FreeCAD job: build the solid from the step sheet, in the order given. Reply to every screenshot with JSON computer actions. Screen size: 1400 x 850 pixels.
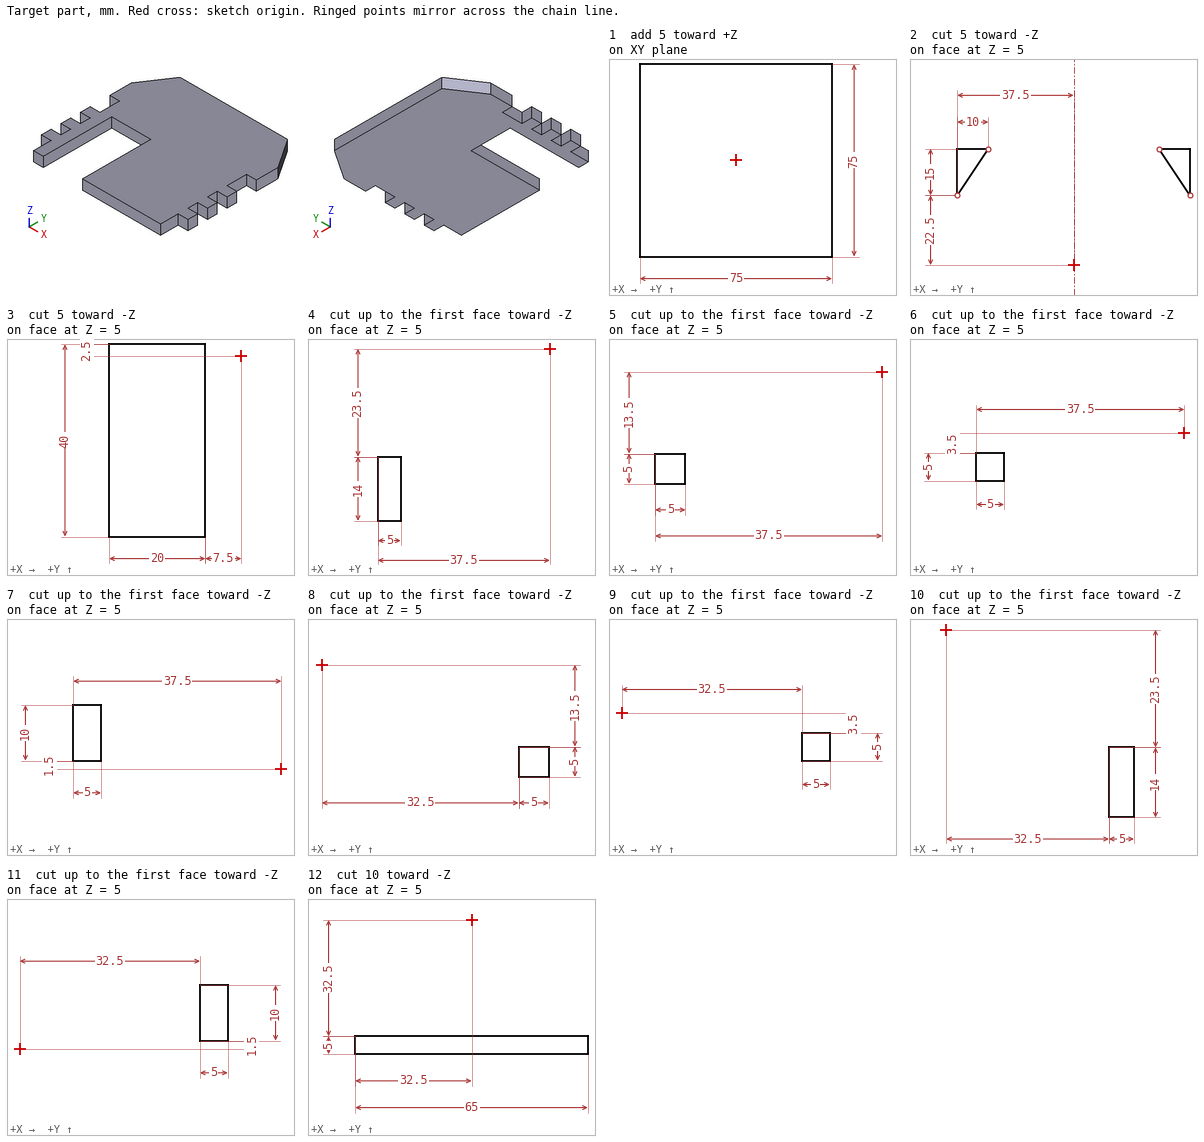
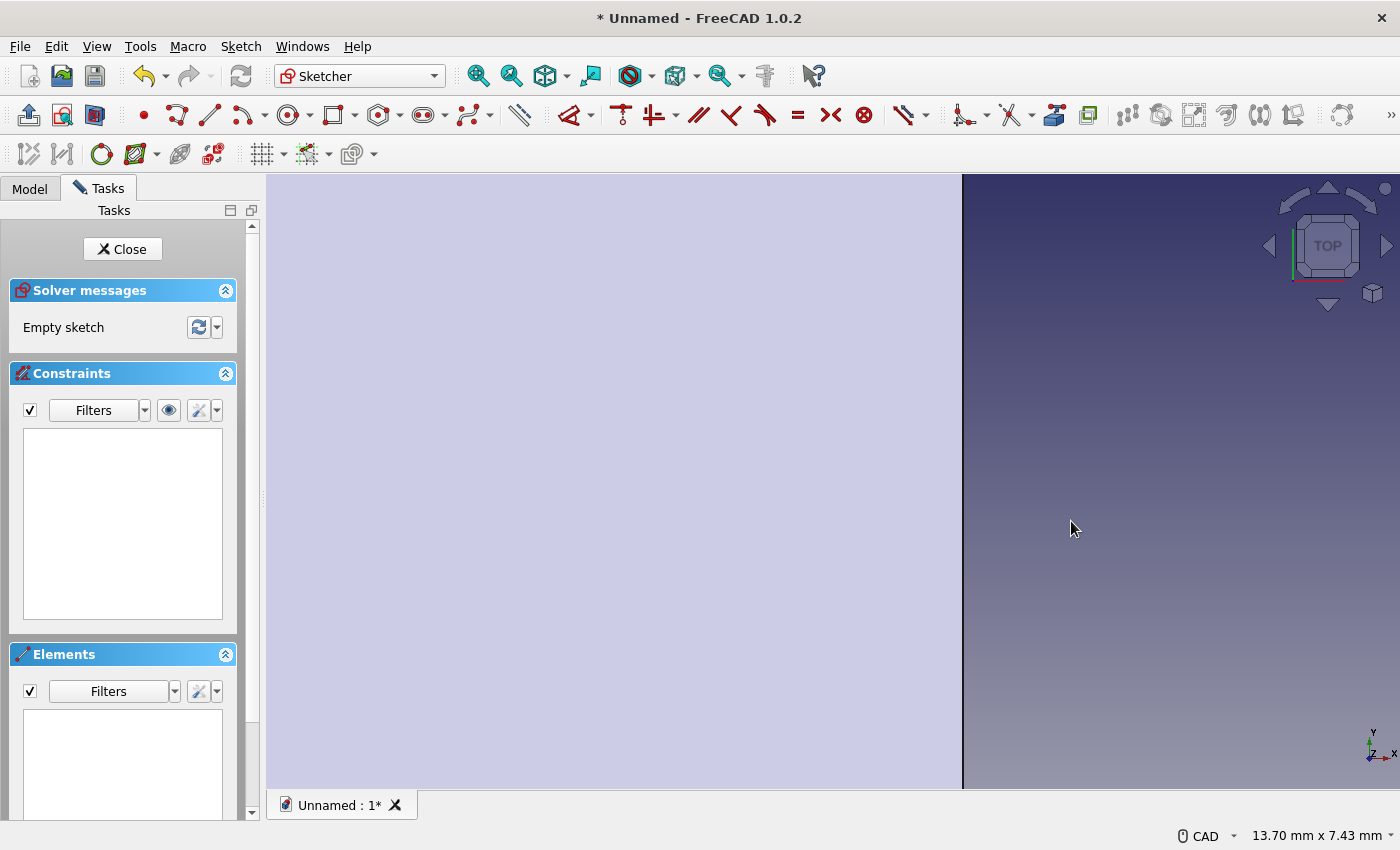
{"action": "key", "text": "g r"}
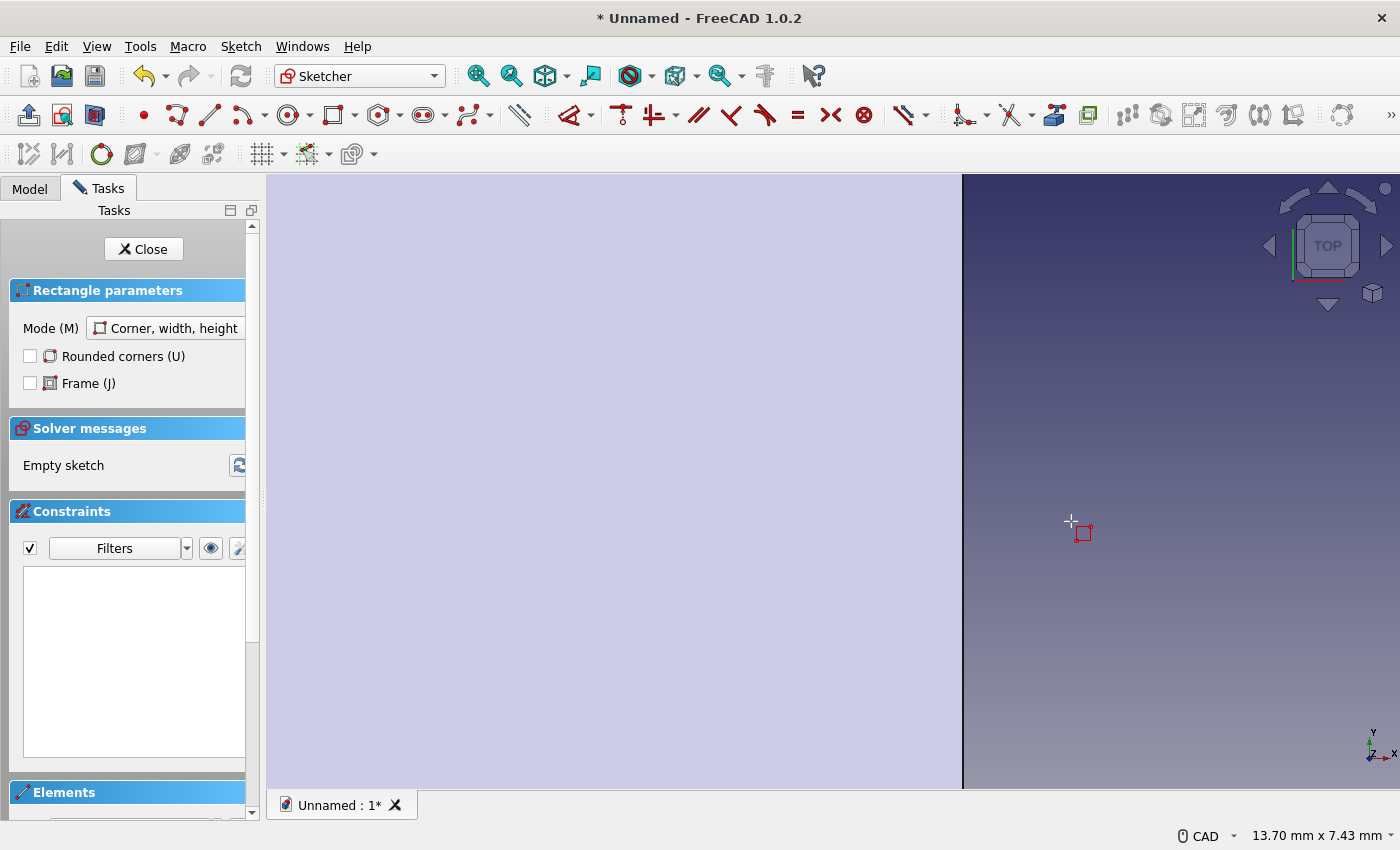
{"action": "left_click", "coordinate": [549, 272]}
{"action": "left_click", "coordinate": [963, 686]}
{"action": "key", "text": "Escape"}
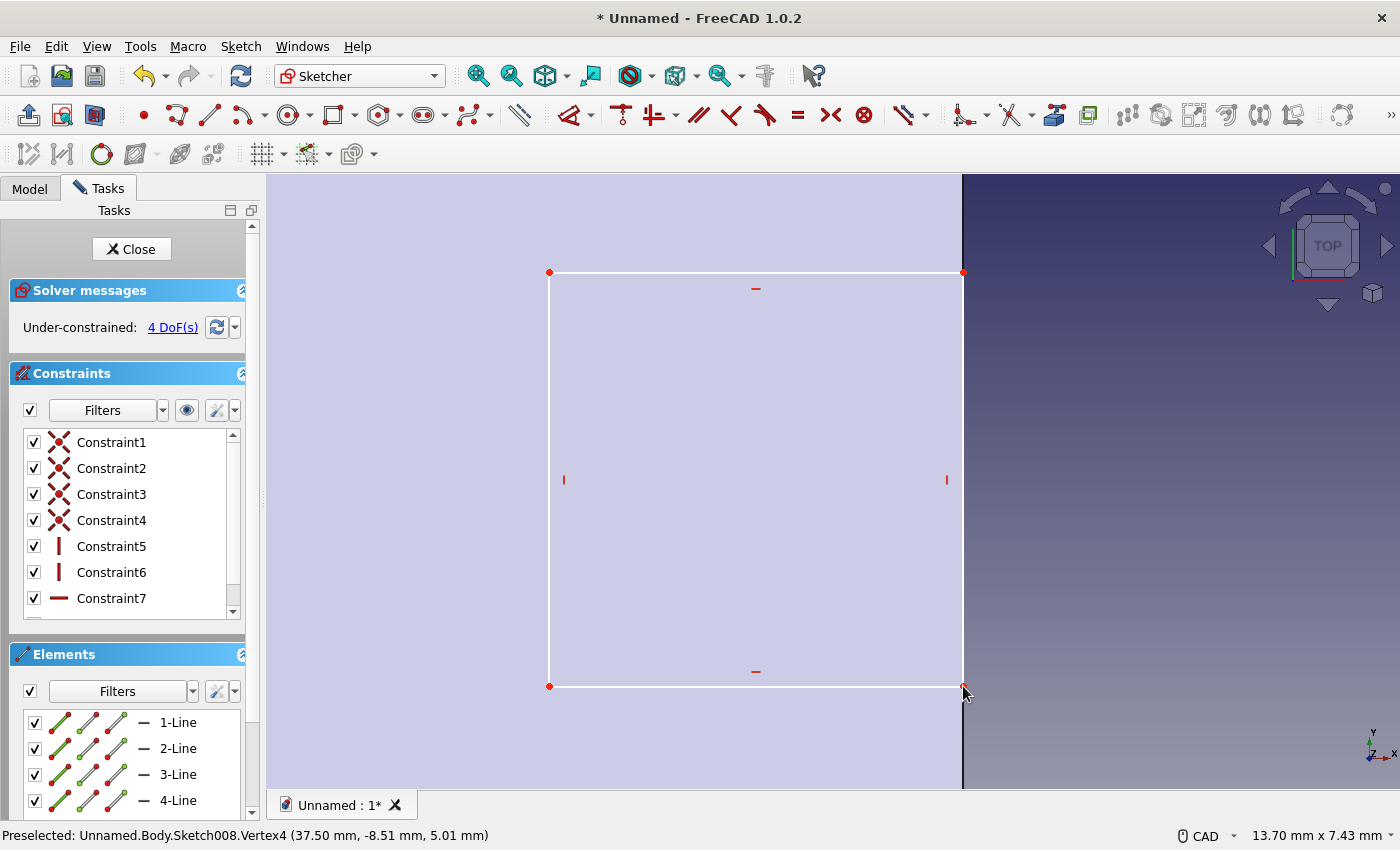
{"action": "left_click", "coordinate": [568, 116]}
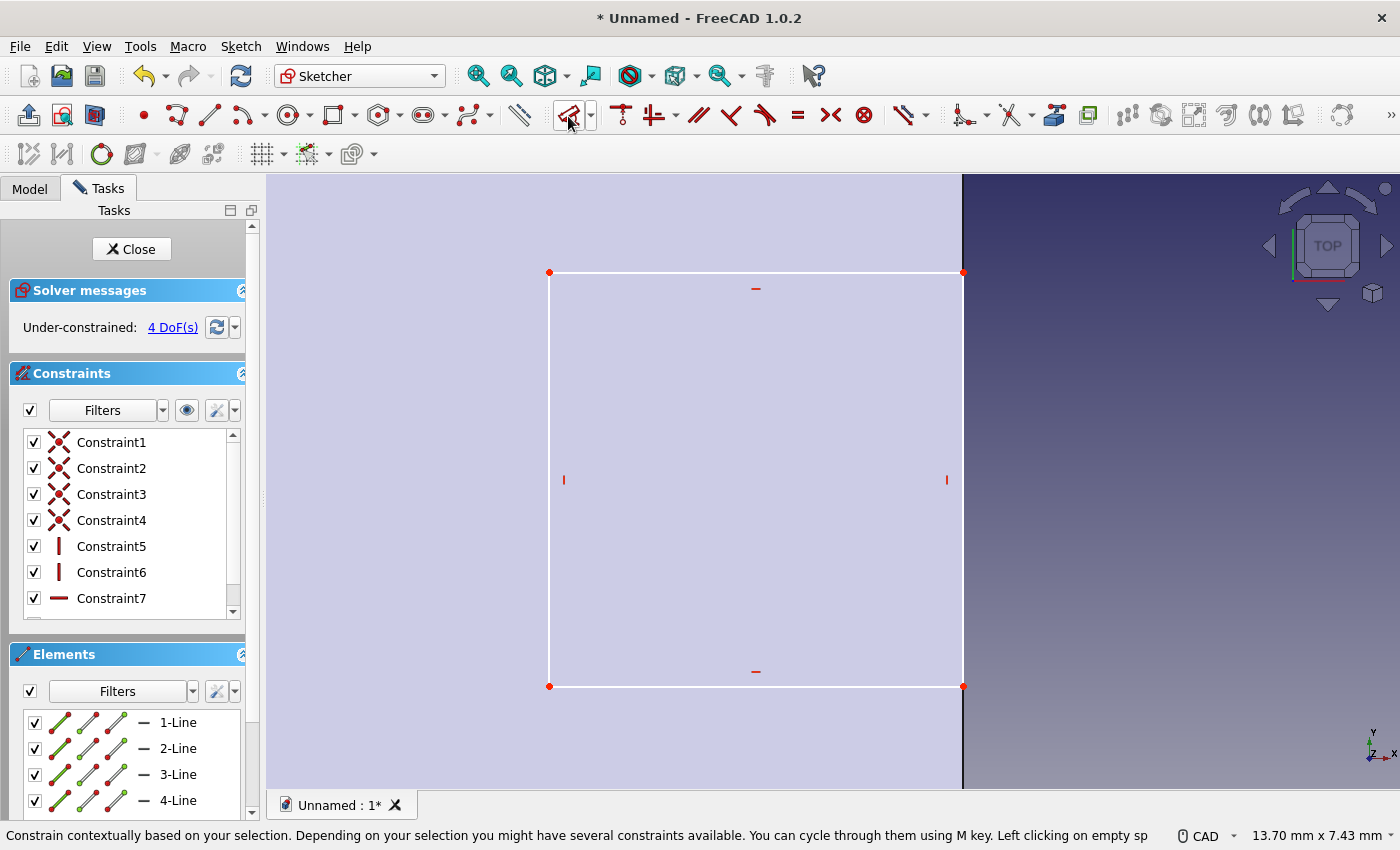
{"action": "left_click", "coordinate": [549, 397]}
{"action": "left_click", "coordinate": [515, 480]}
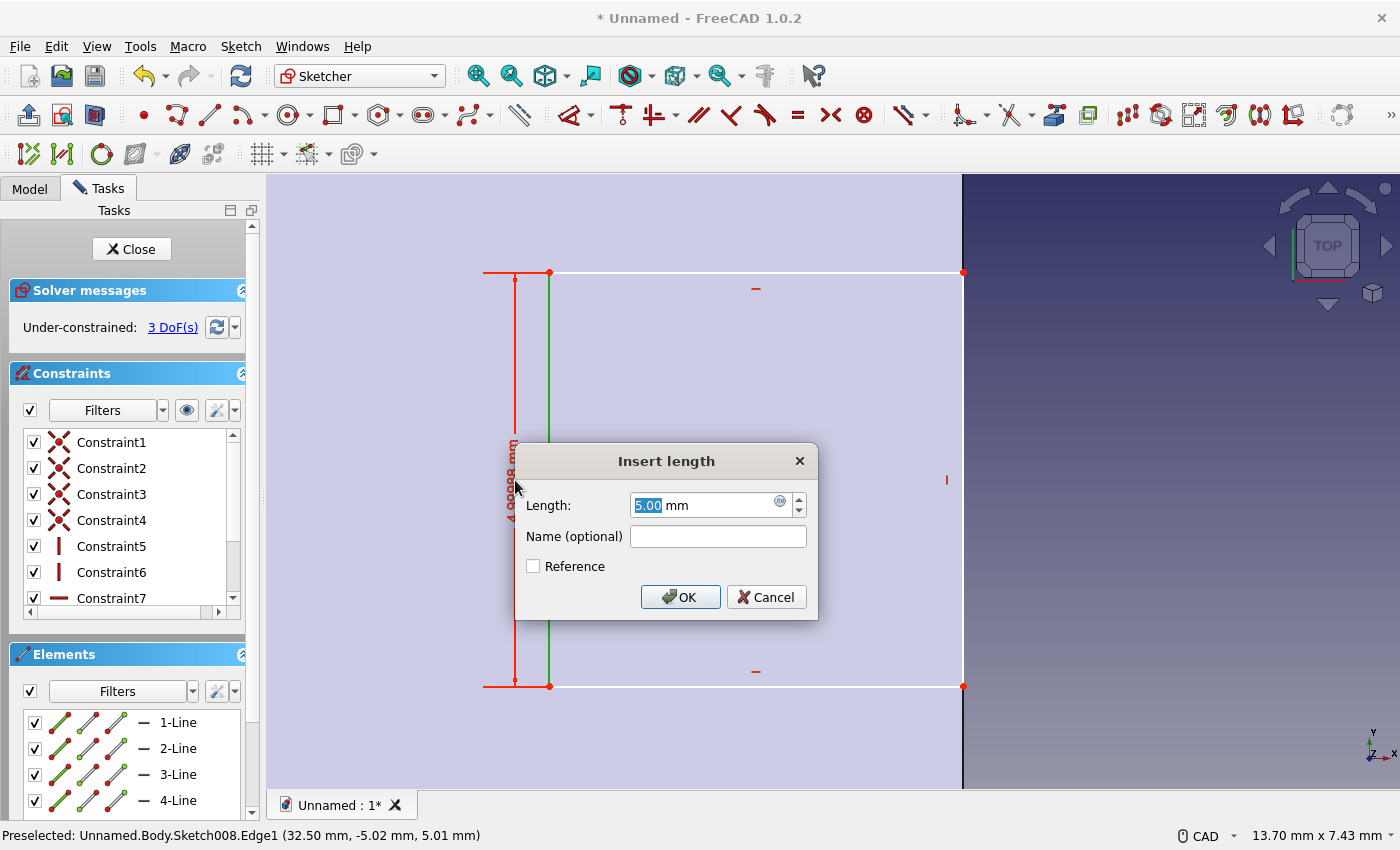
{"action": "type", "text": "5"}
{"action": "key", "text": "Return"}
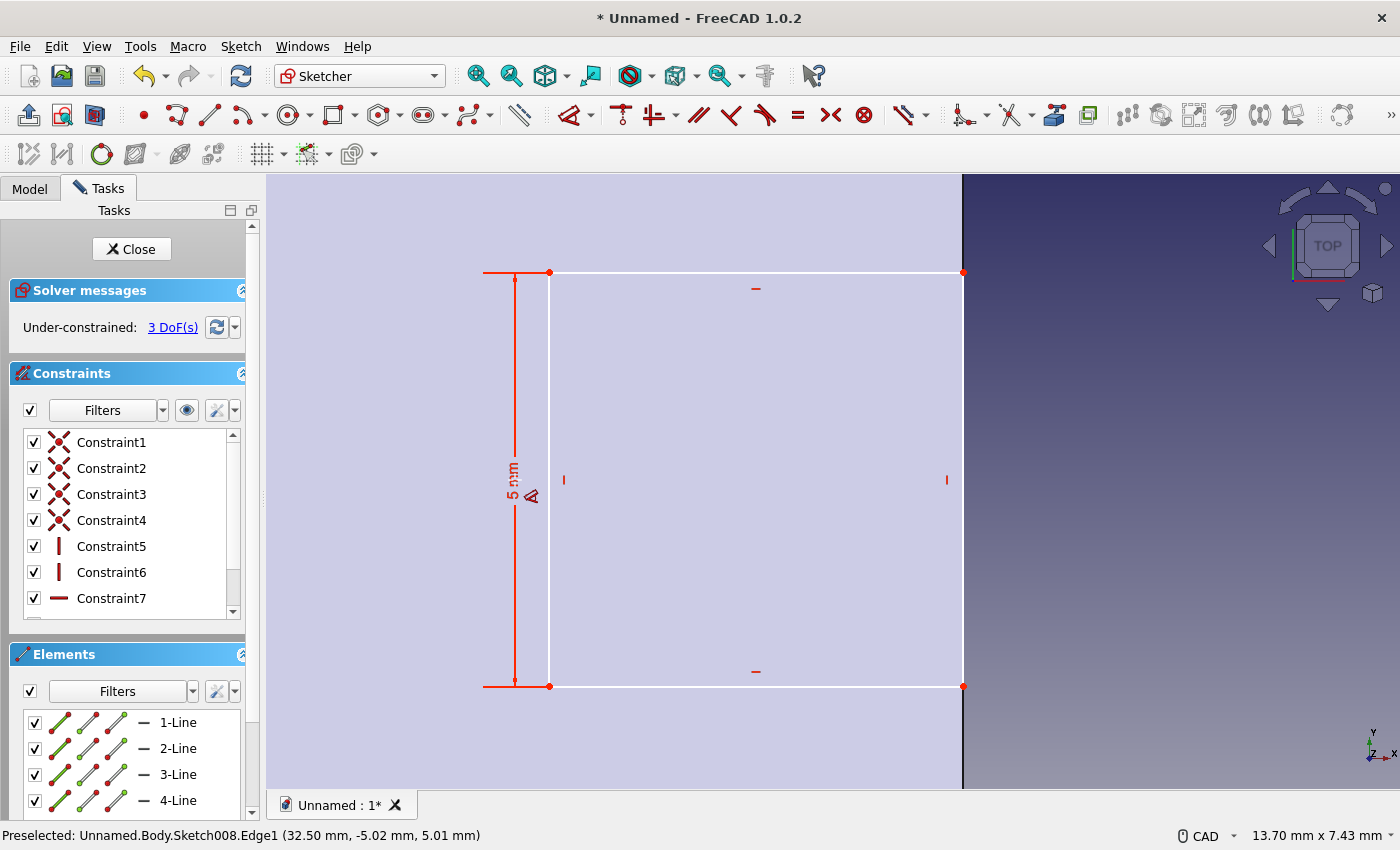
{"action": "left_click", "coordinate": [673, 687]}
{"action": "left_click", "coordinate": [756, 721]}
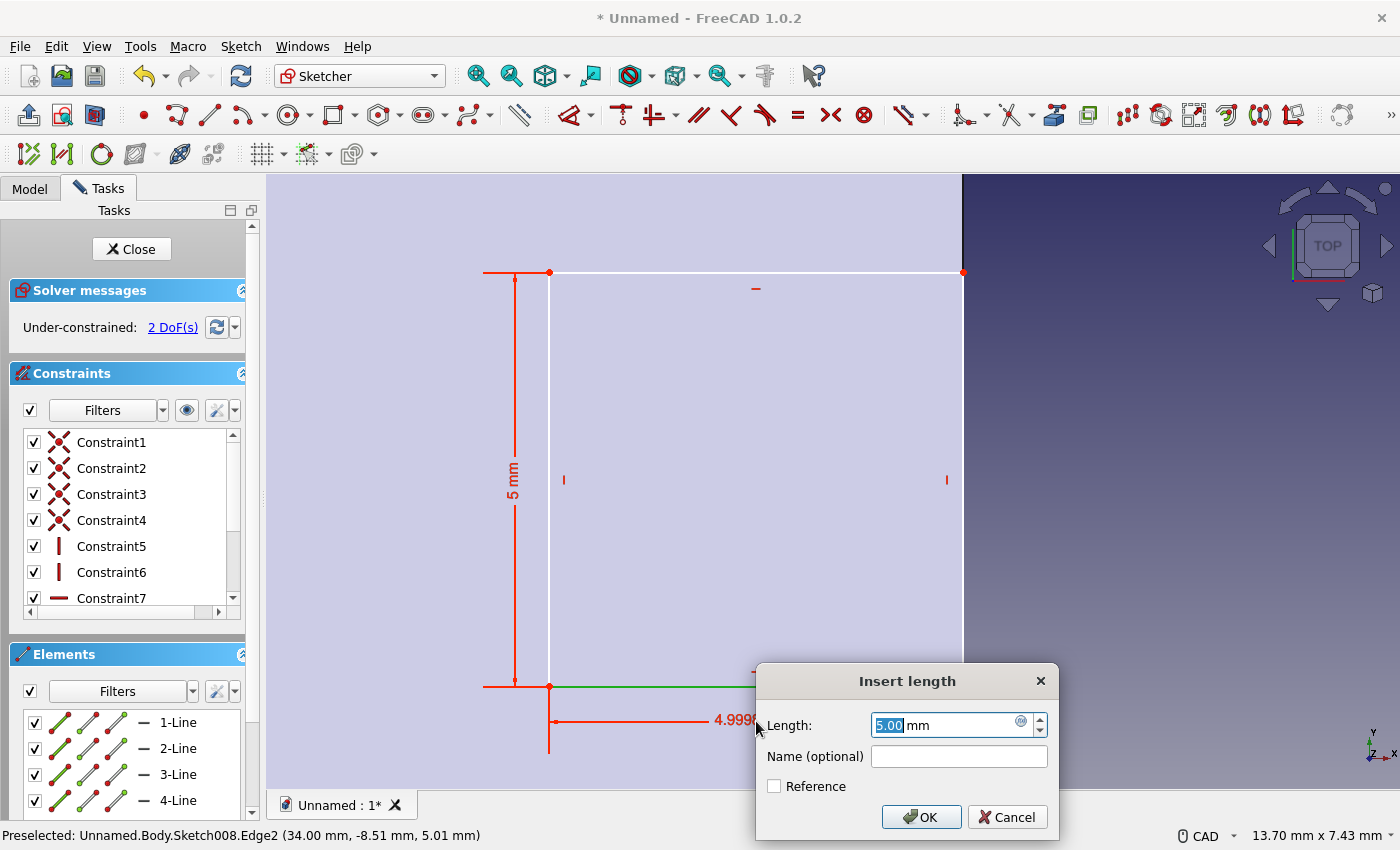
{"action": "type", "text": "5"}
{"action": "key", "text": "Return"}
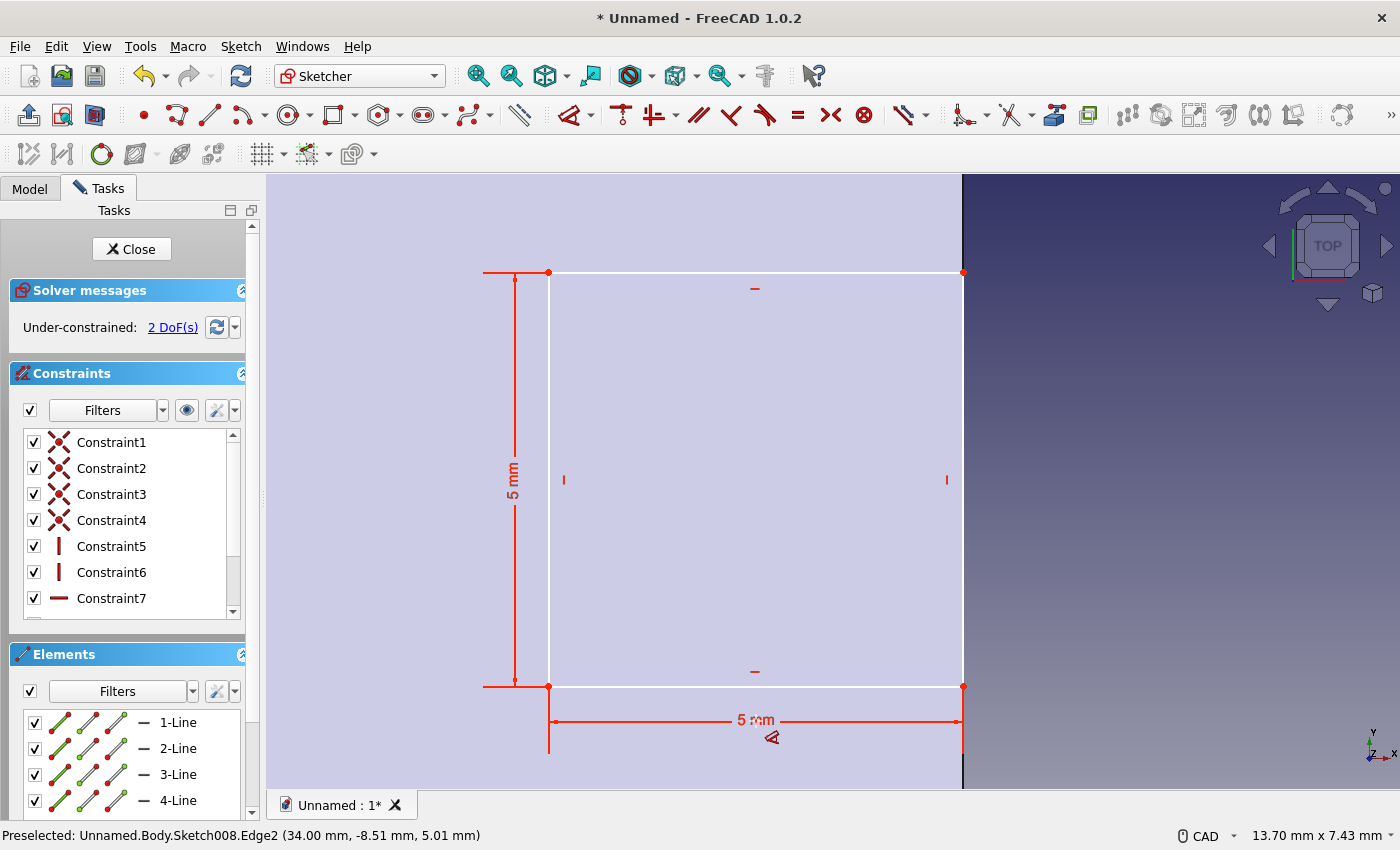
{"action": "left_click", "coordinate": [549, 273]}
{"action": "left_click", "coordinate": [583, 237]}